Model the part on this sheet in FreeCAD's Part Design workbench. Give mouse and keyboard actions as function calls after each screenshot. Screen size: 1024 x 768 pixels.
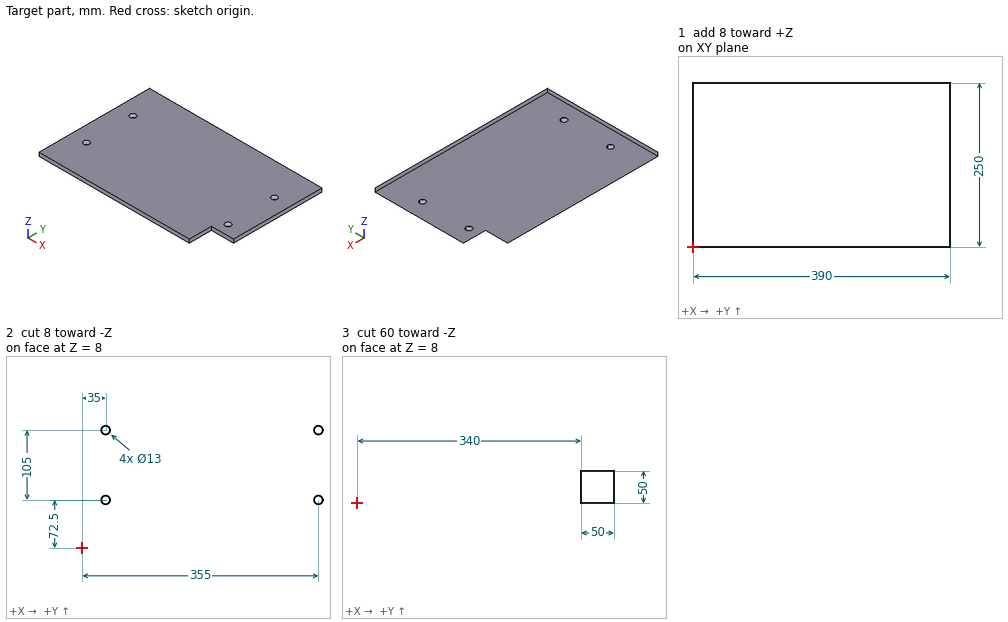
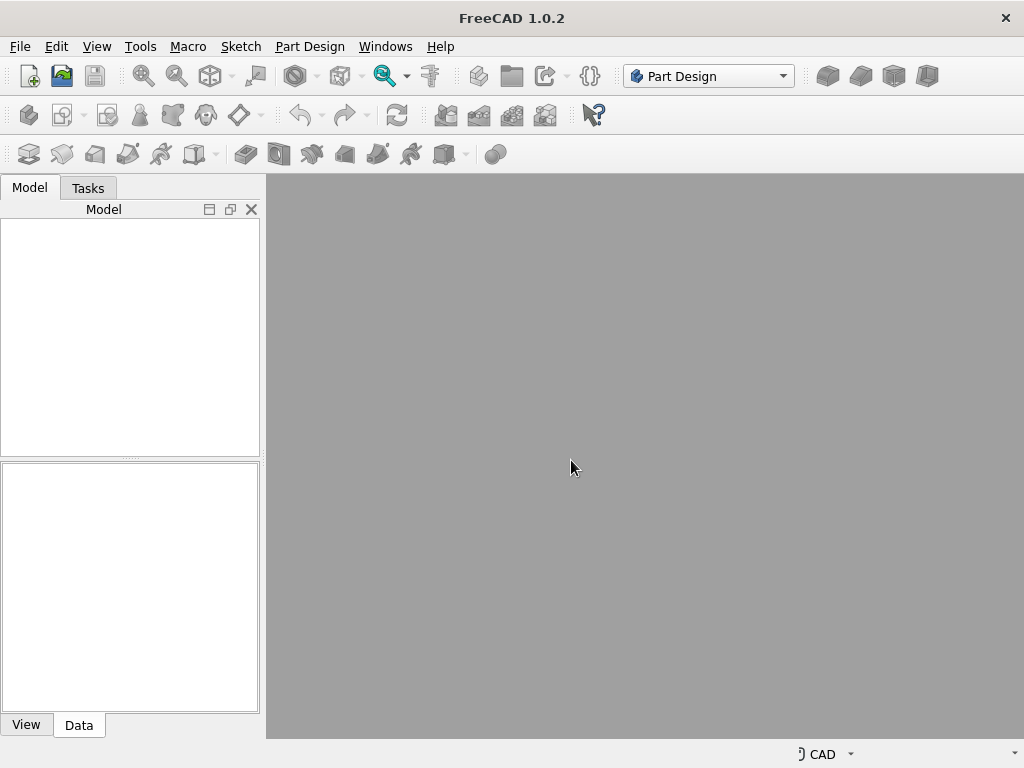
key(ctrl+n)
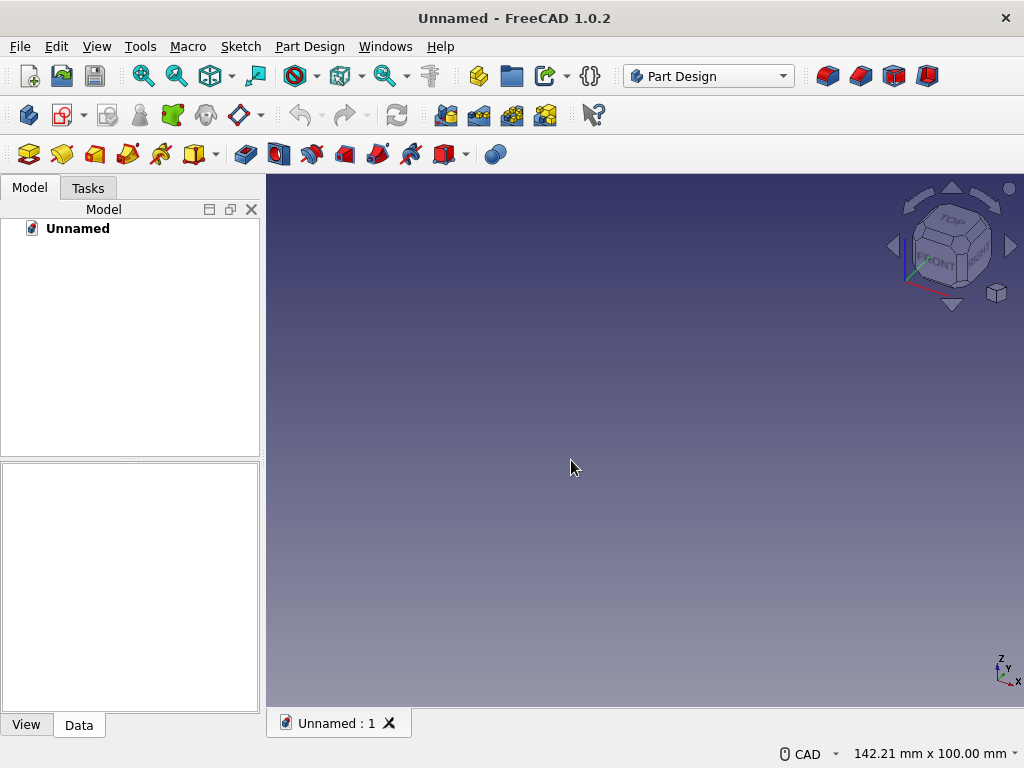
click(62, 116)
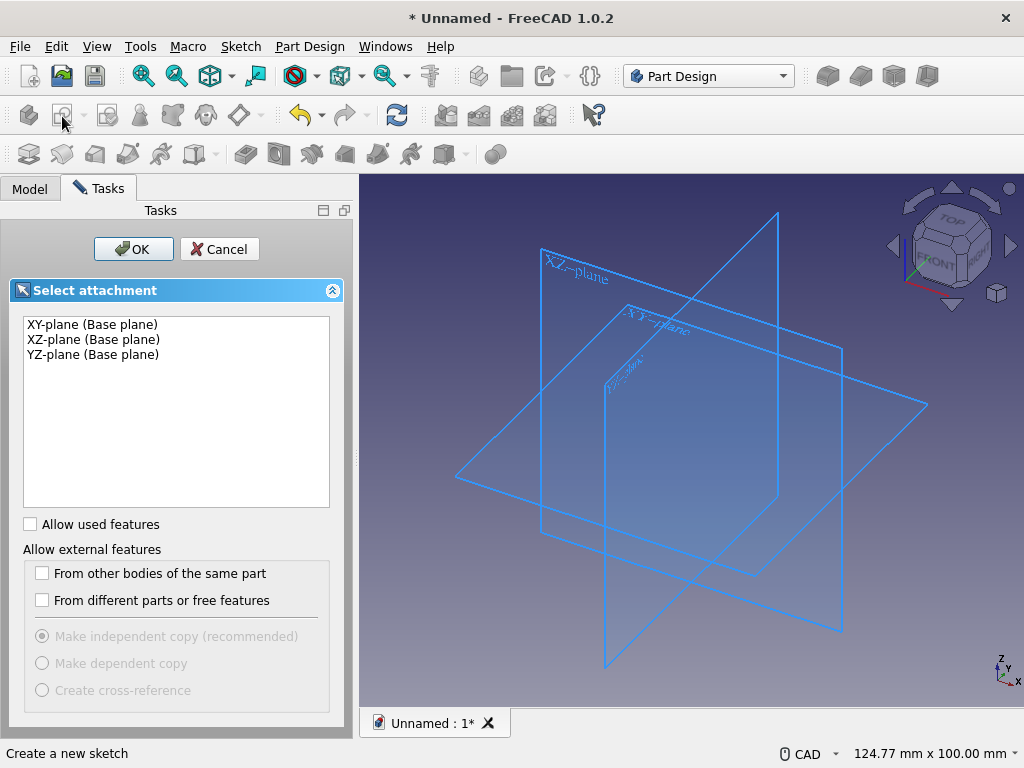
click(84, 324)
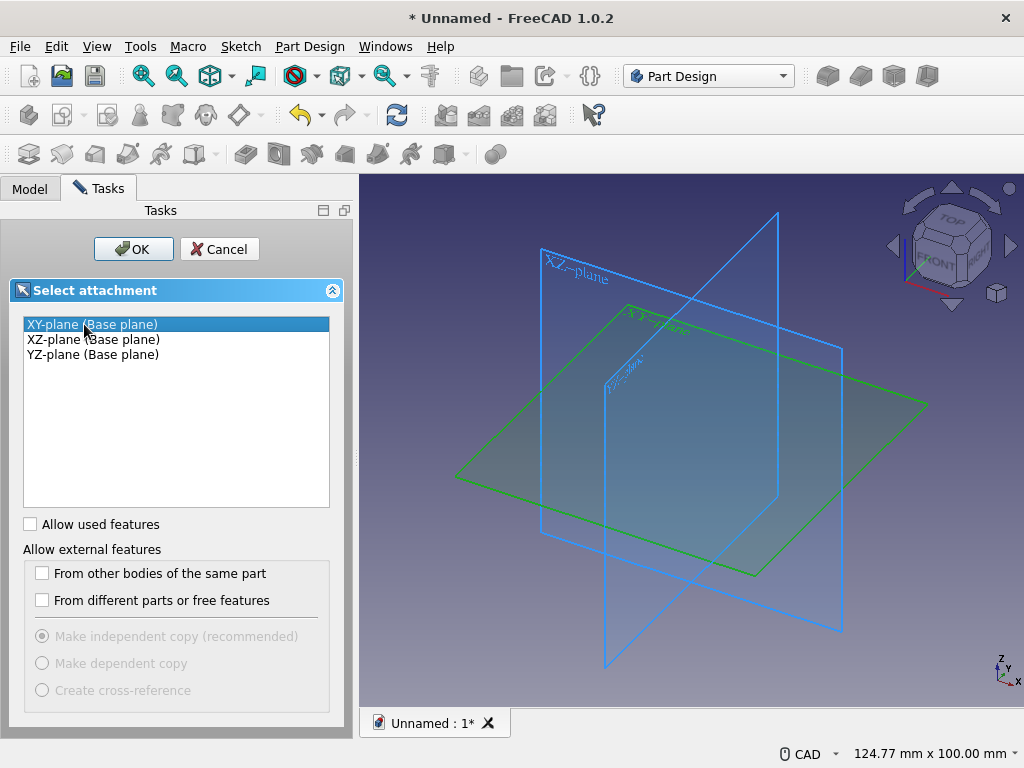
click(134, 249)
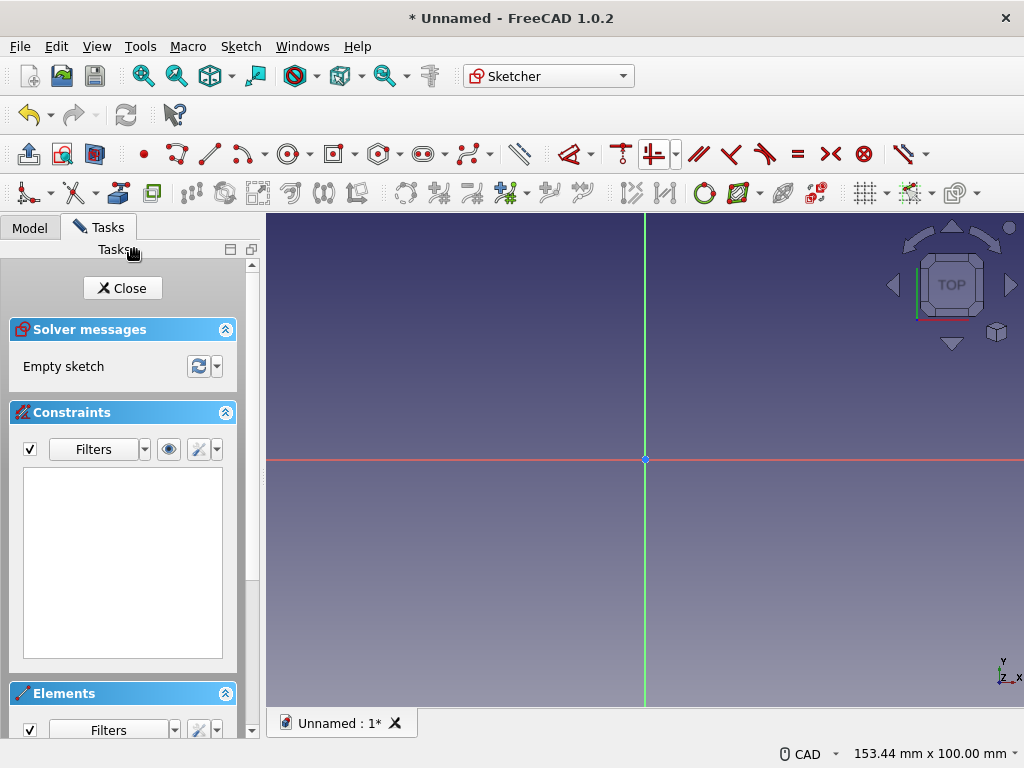
scroll(315, 616, down, 8)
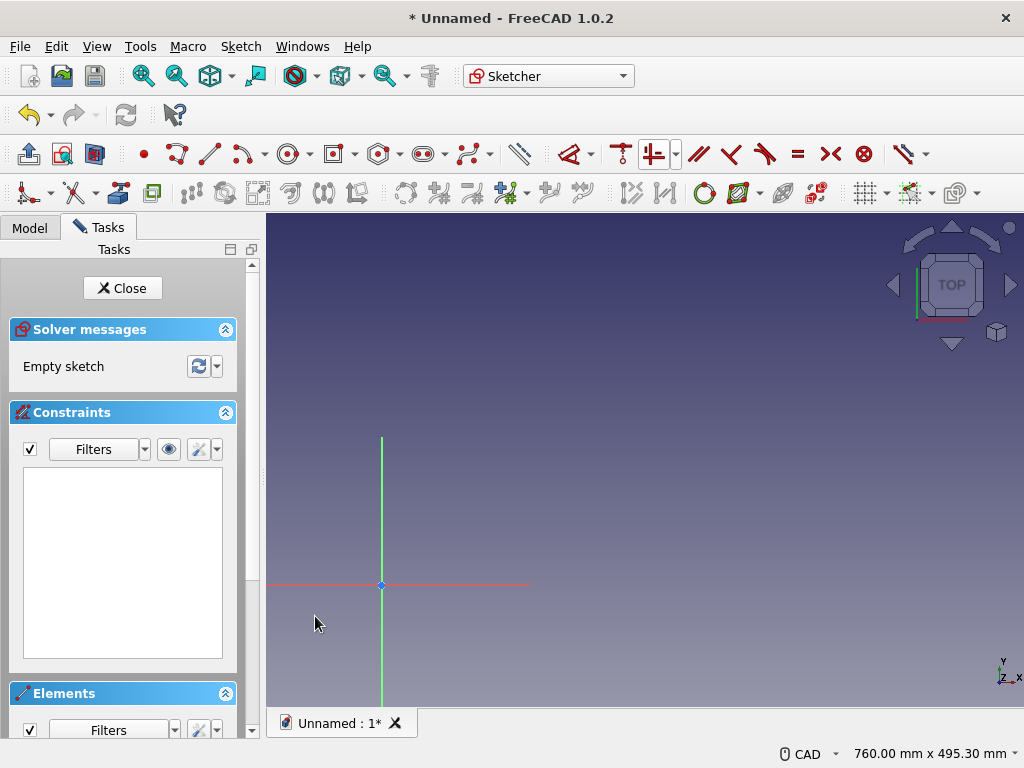
click(354, 154)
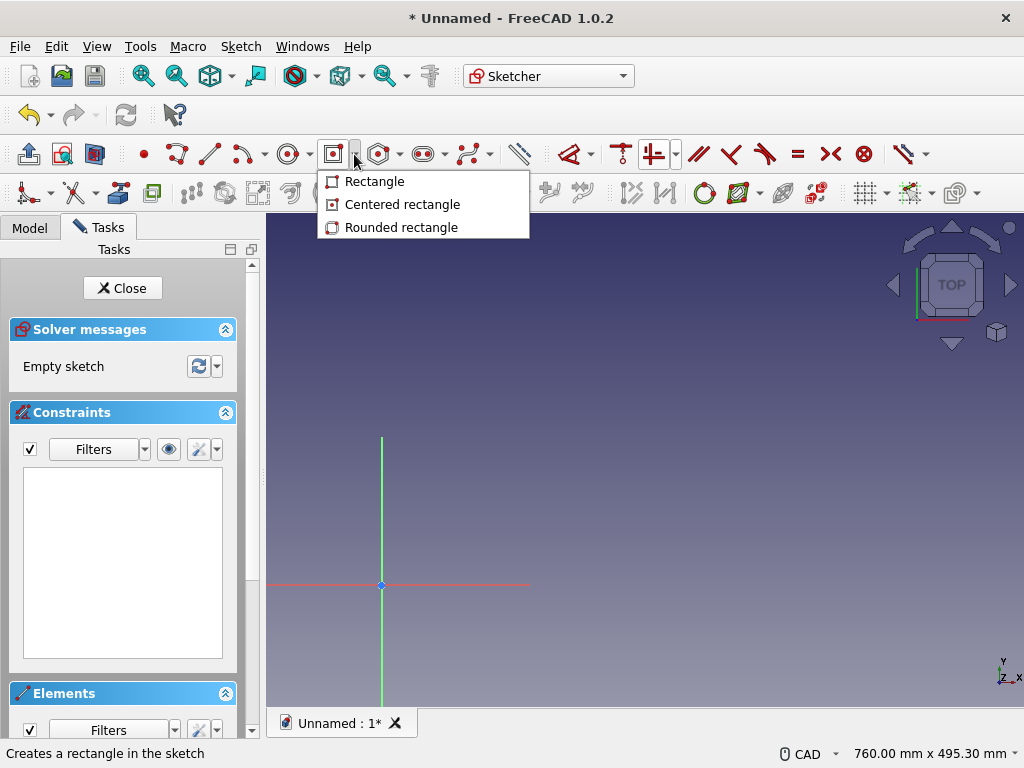
click(424, 182)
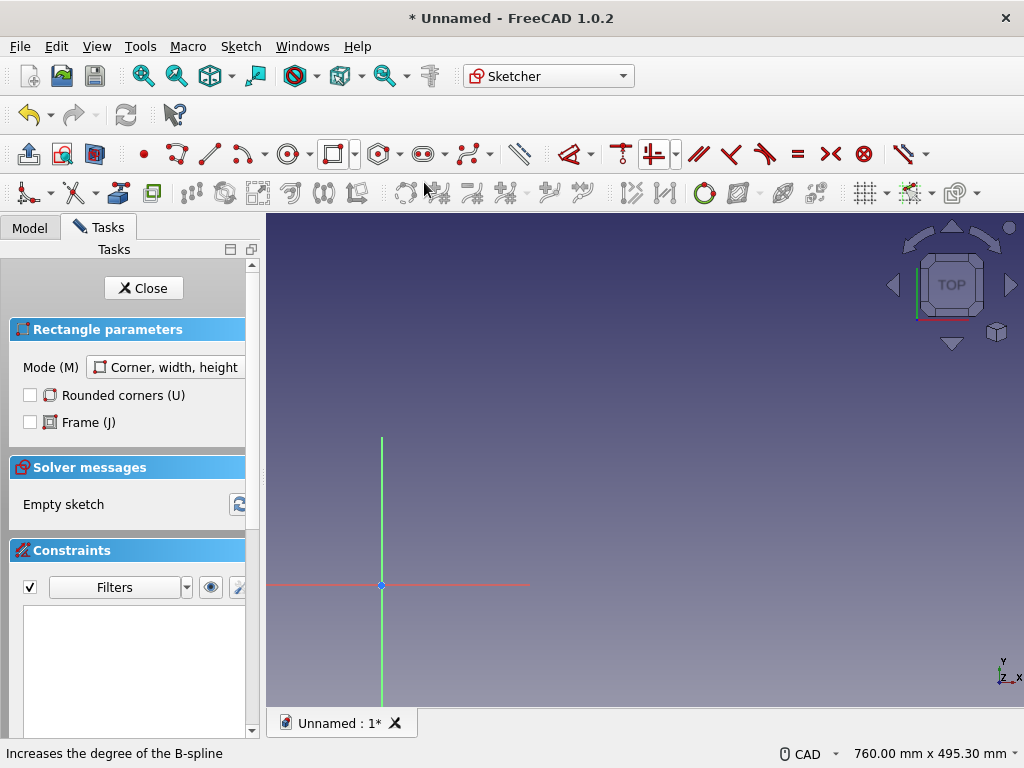
click(382, 585)
move(771, 336)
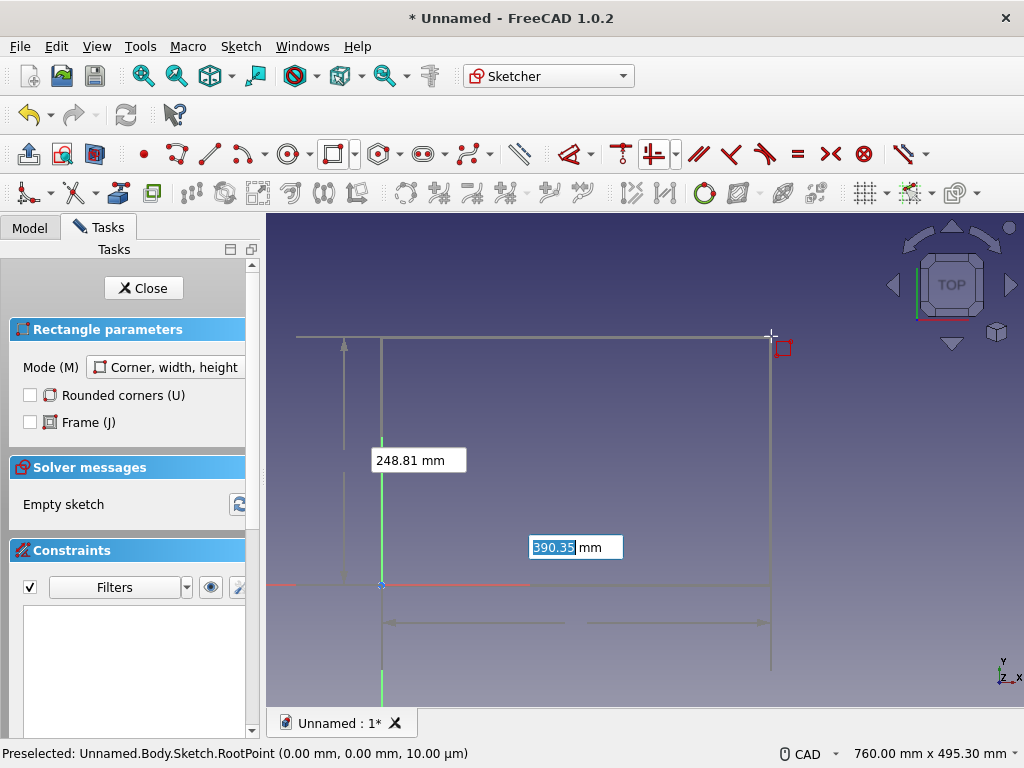
text(390)
key(Tab)
text(250)
key(Return)
key(Escape)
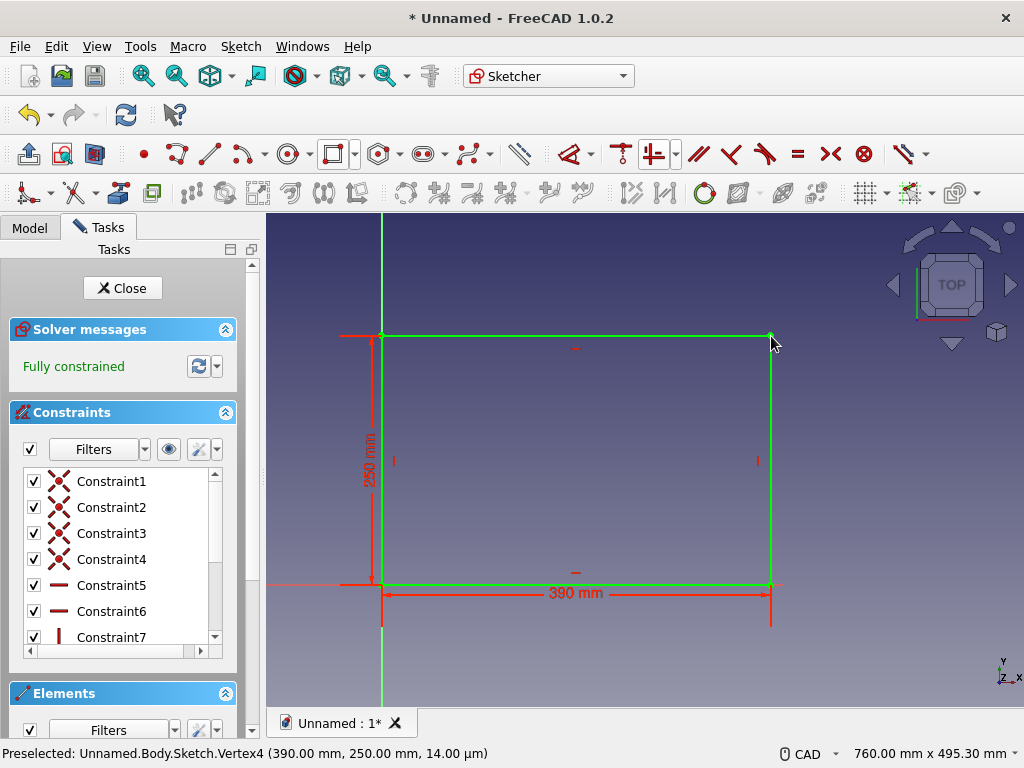
click(123, 288)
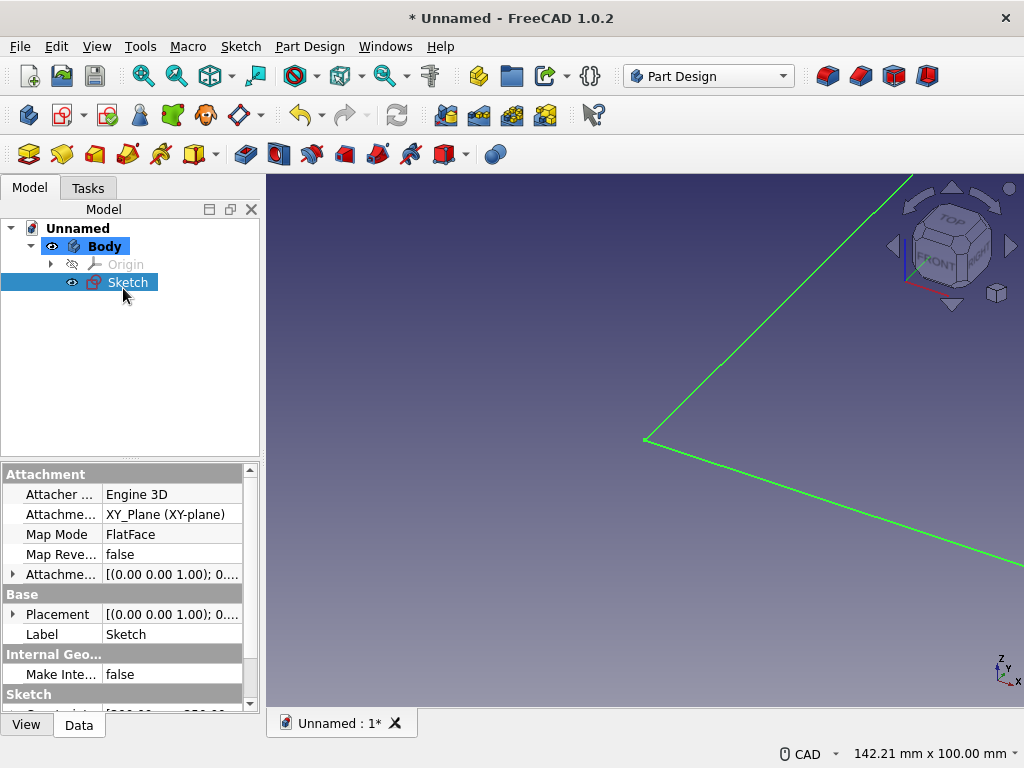
click(29, 154)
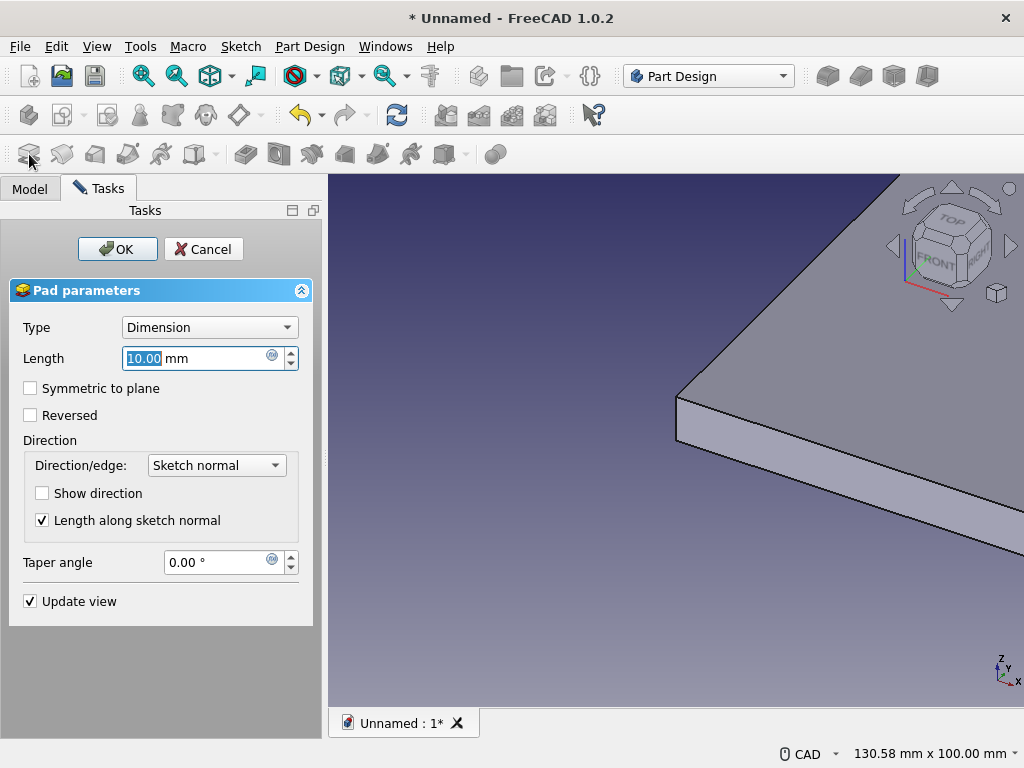
text(8)
key(Tab)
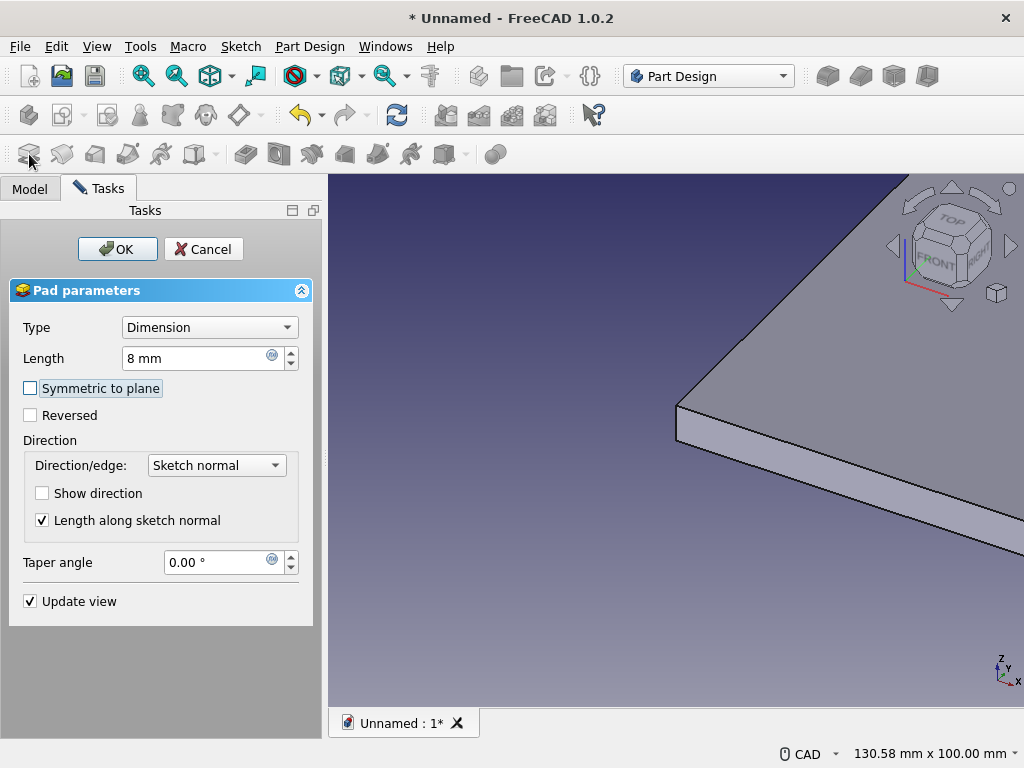
click(118, 249)